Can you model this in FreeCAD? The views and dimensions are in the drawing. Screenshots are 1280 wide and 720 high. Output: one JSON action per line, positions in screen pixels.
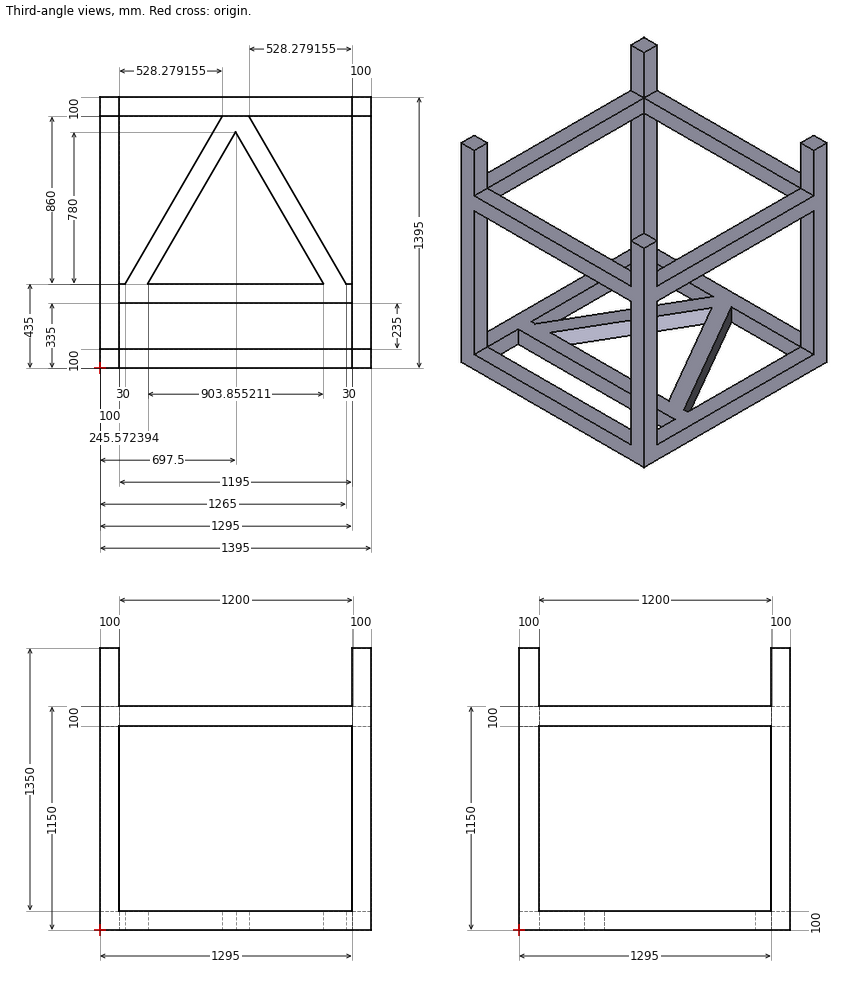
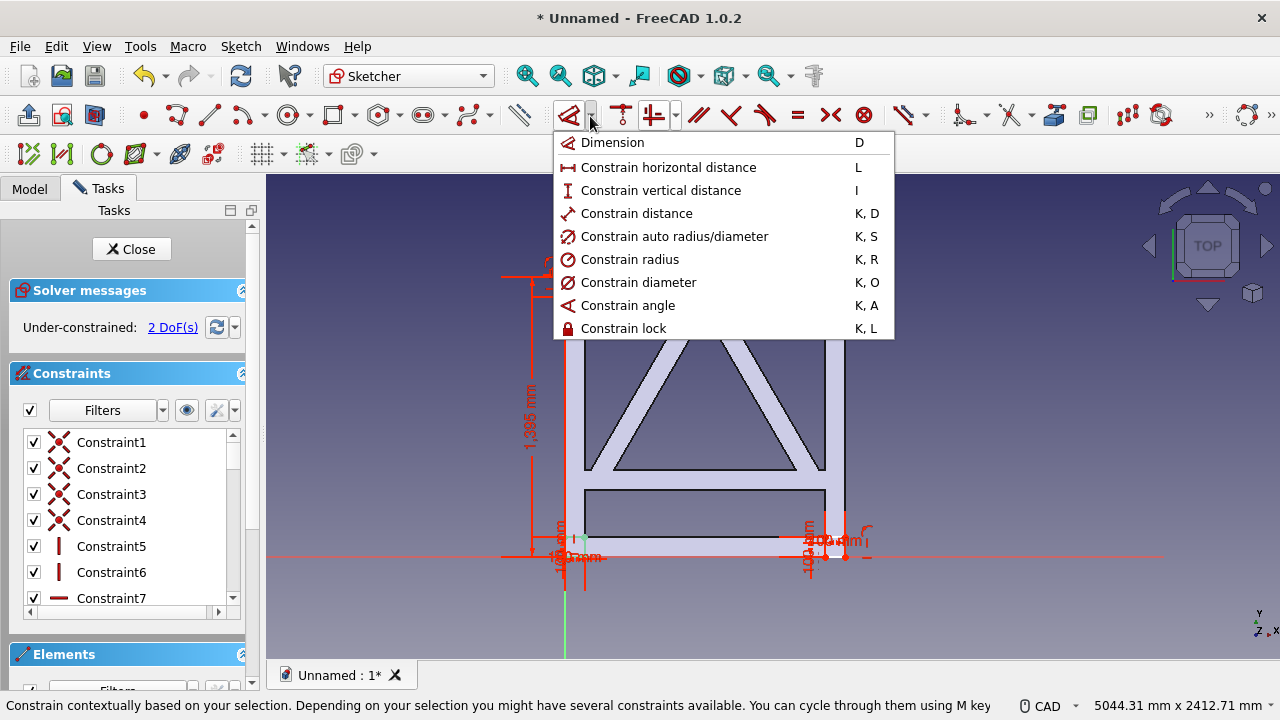
{"action": "left_click", "coordinate": [724, 190]}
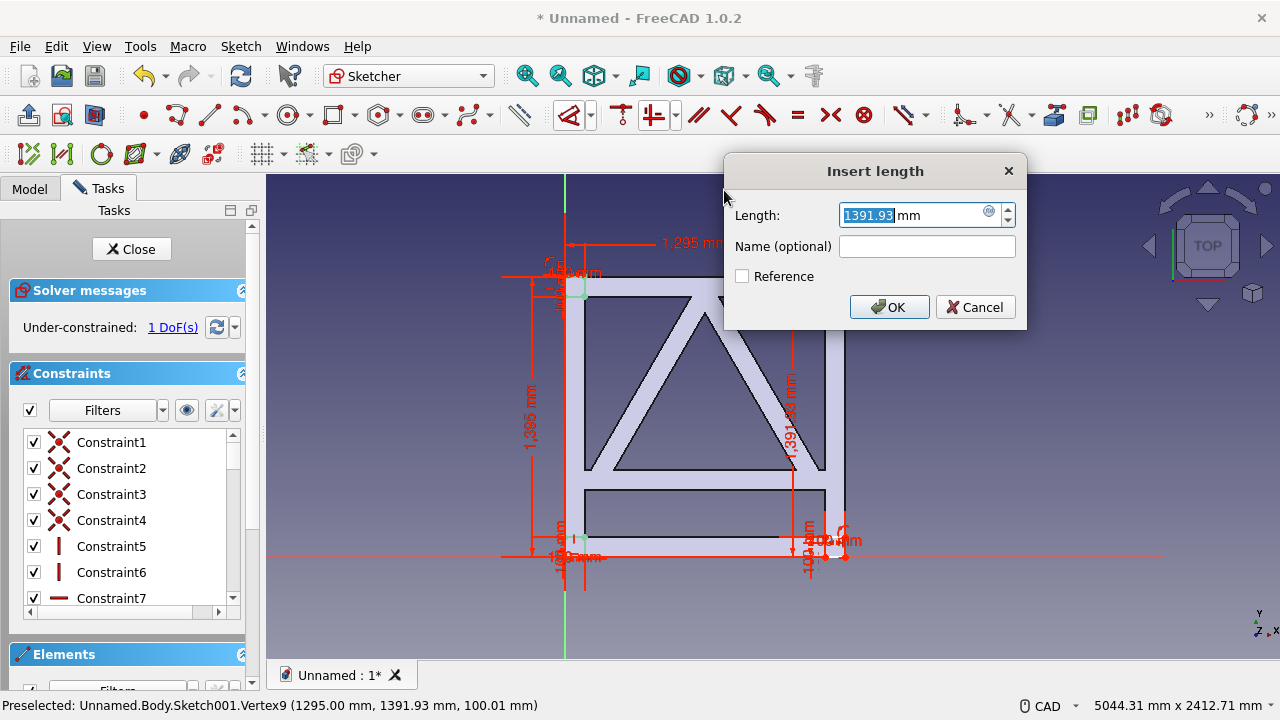
{"action": "type", "text": "1395"}
{"action": "key", "text": "Return"}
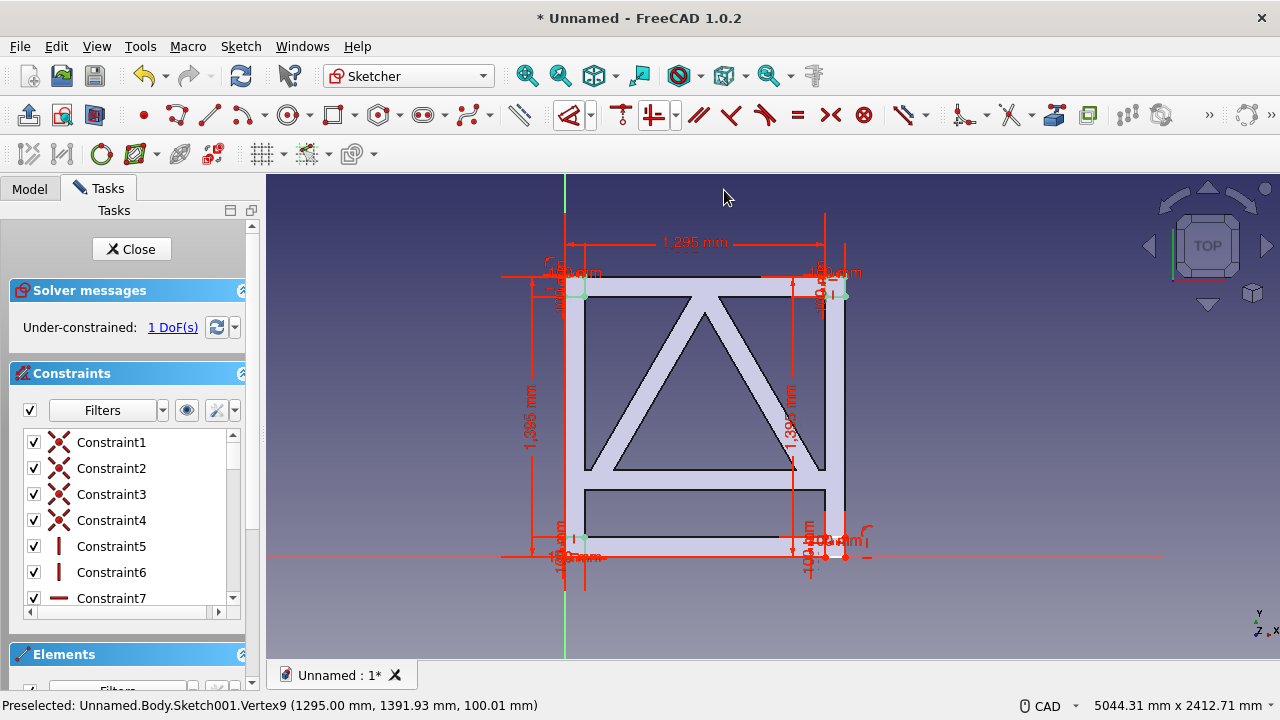
{"action": "left_click", "coordinate": [825, 537]}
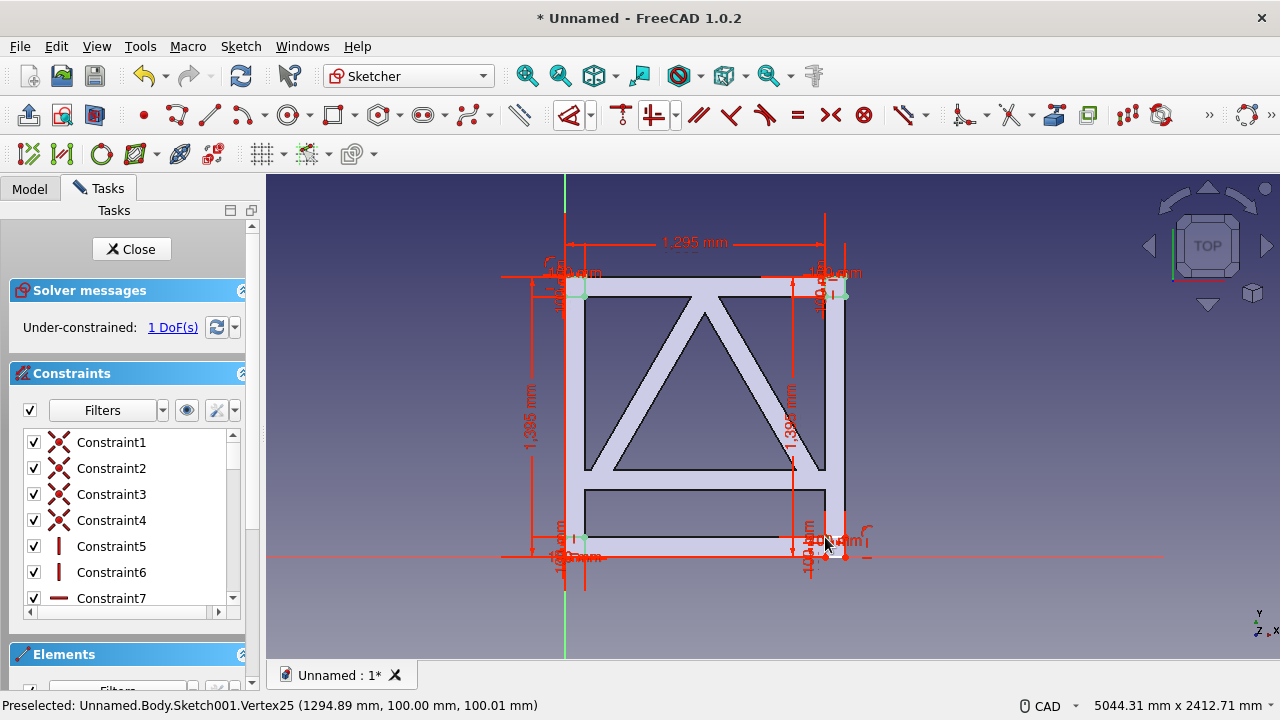
{"action": "left_click", "coordinate": [590, 116]}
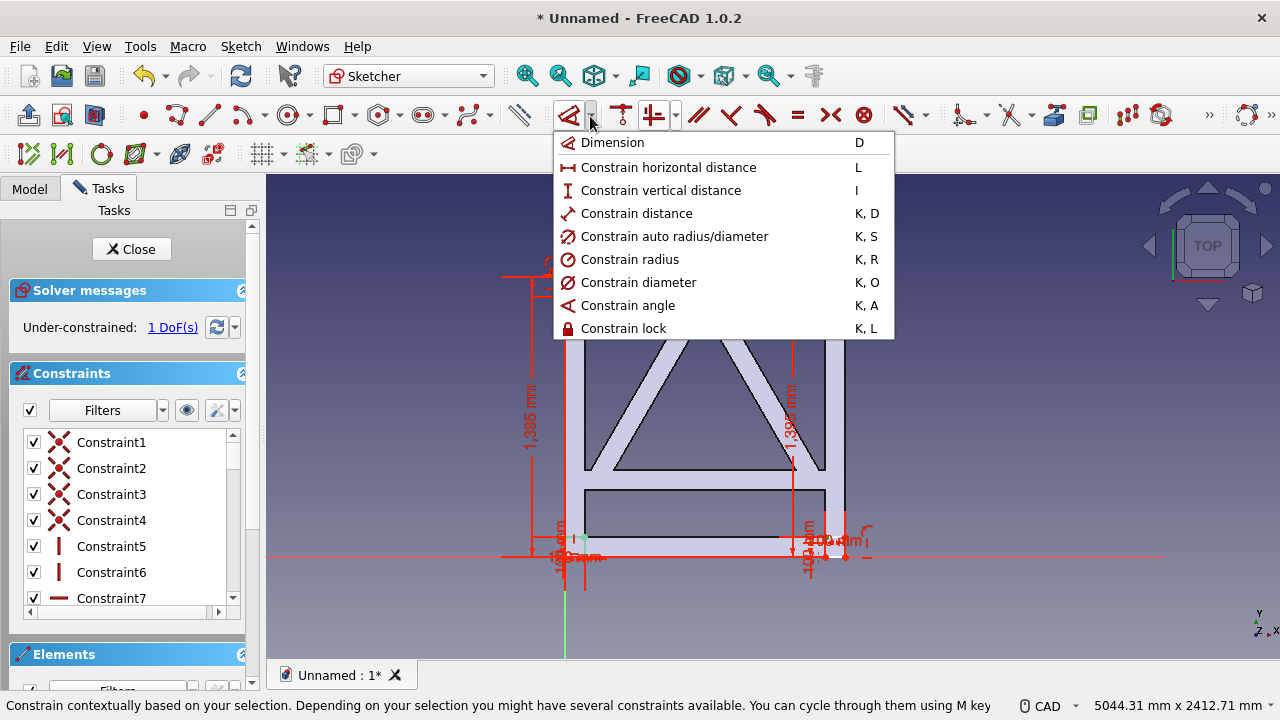
{"action": "left_click", "coordinate": [724, 168]}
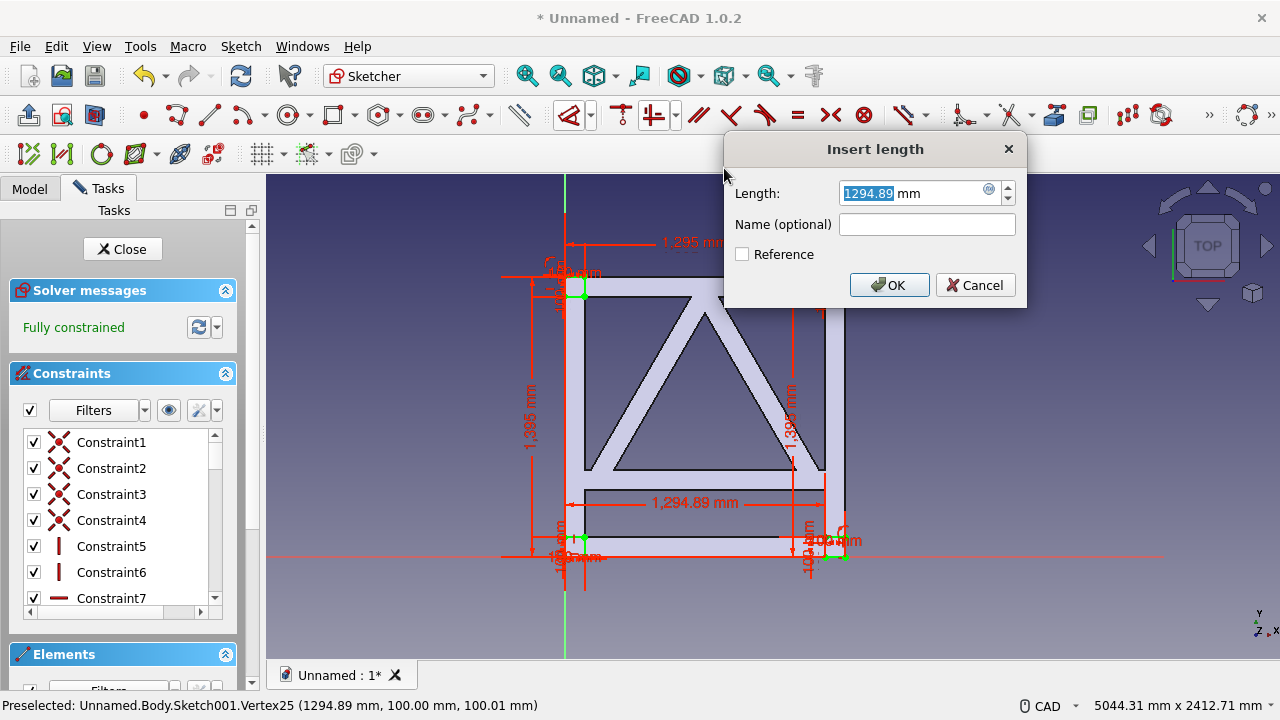
{"action": "type", "text": "1295"}
{"action": "key", "text": "Return"}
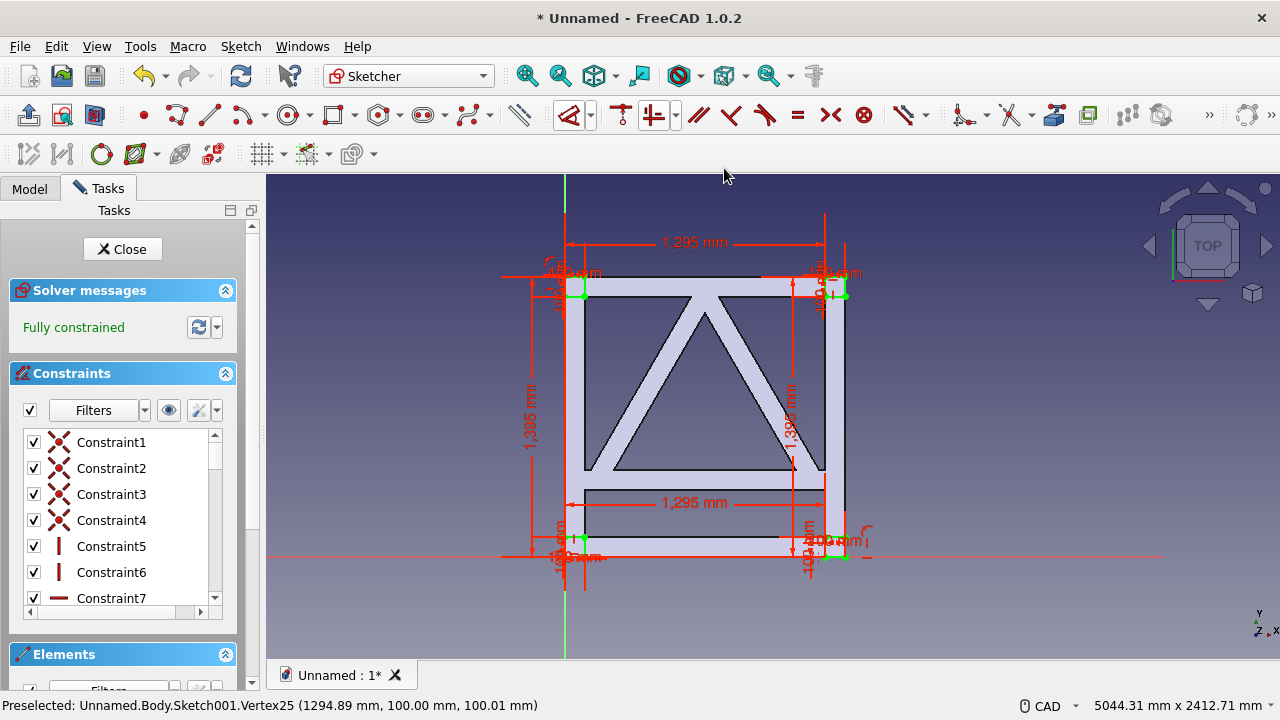
{"action": "left_click", "coordinate": [123, 249]}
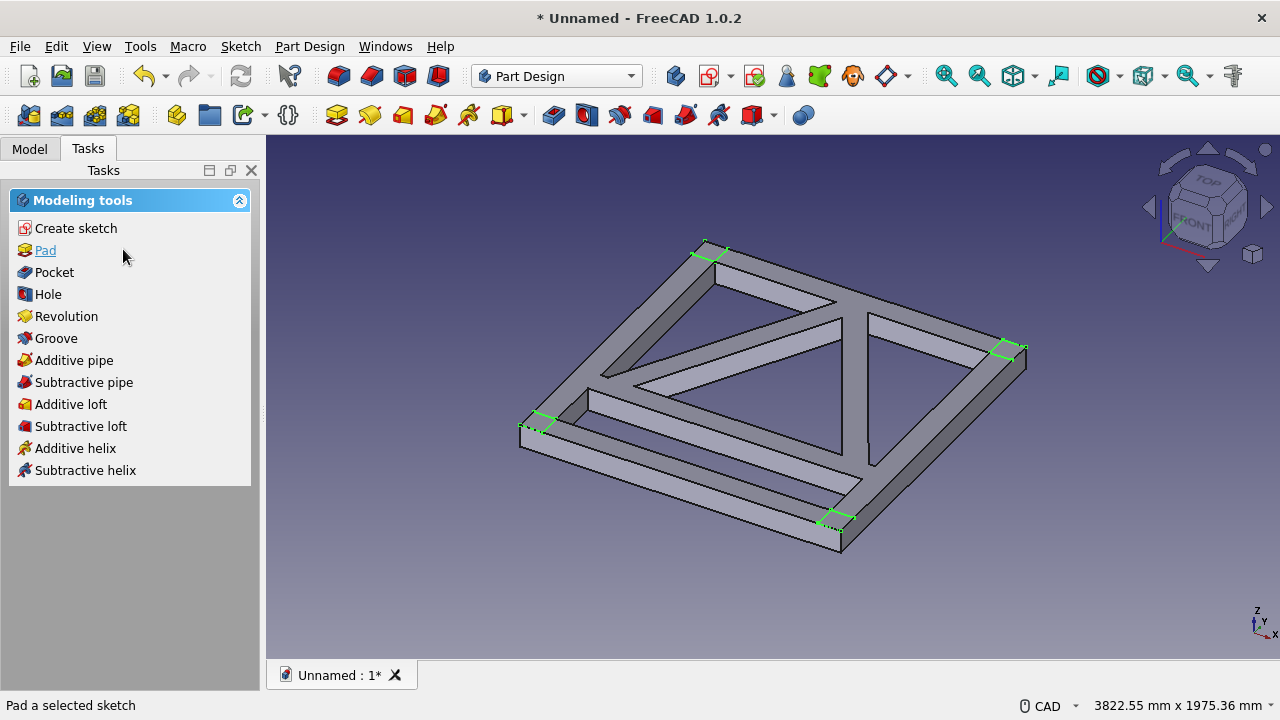
{"action": "left_click", "coordinate": [337, 116]}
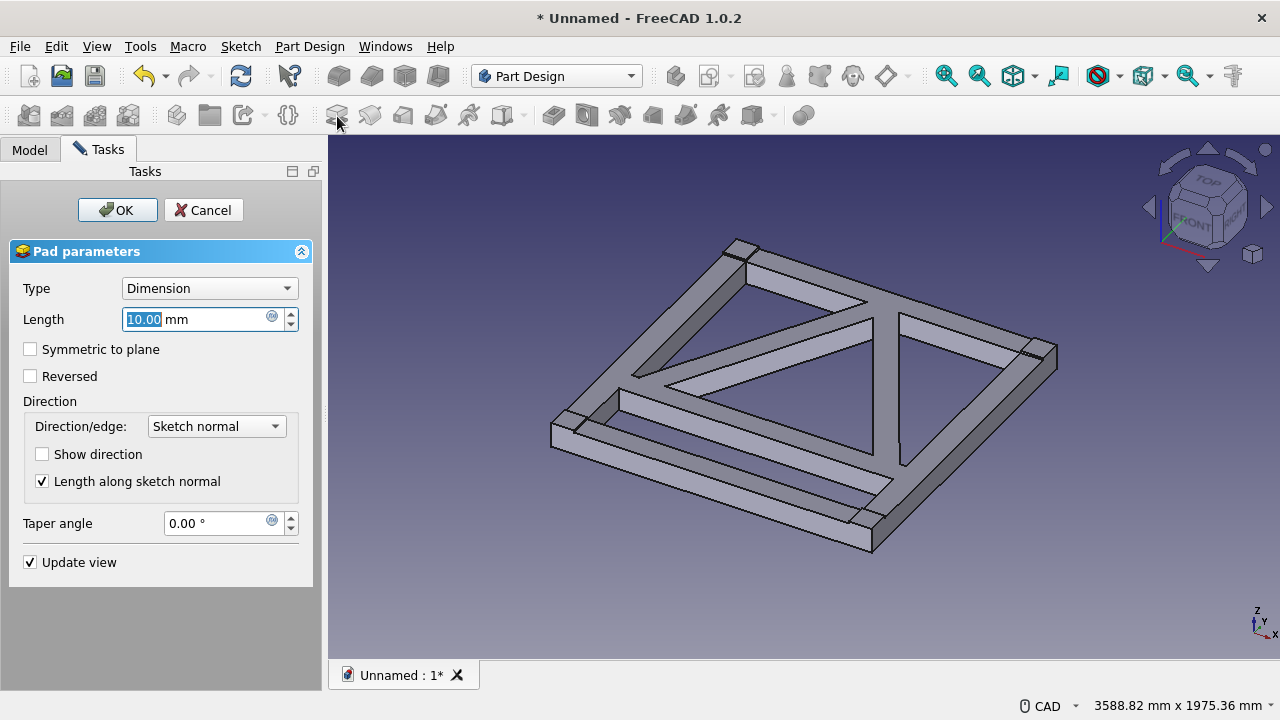
{"action": "type", "text": "1350"}
{"action": "key", "text": "Tab"}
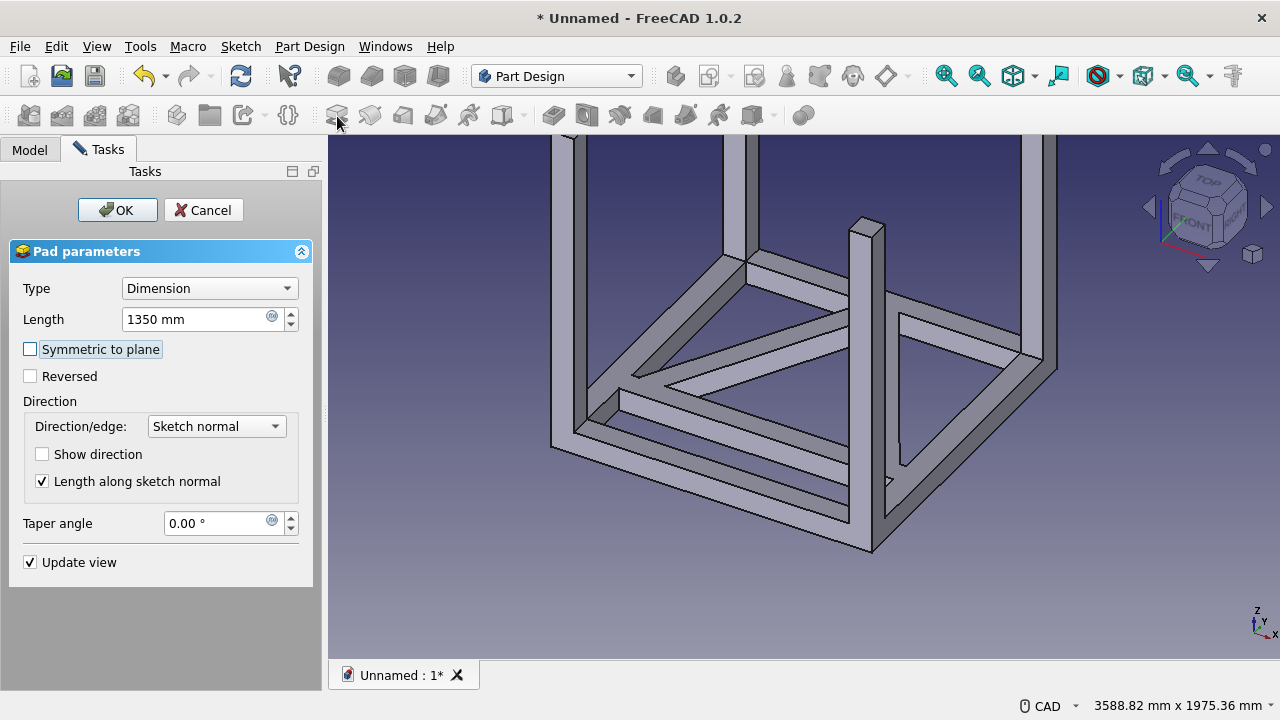
{"action": "left_click", "coordinate": [118, 210]}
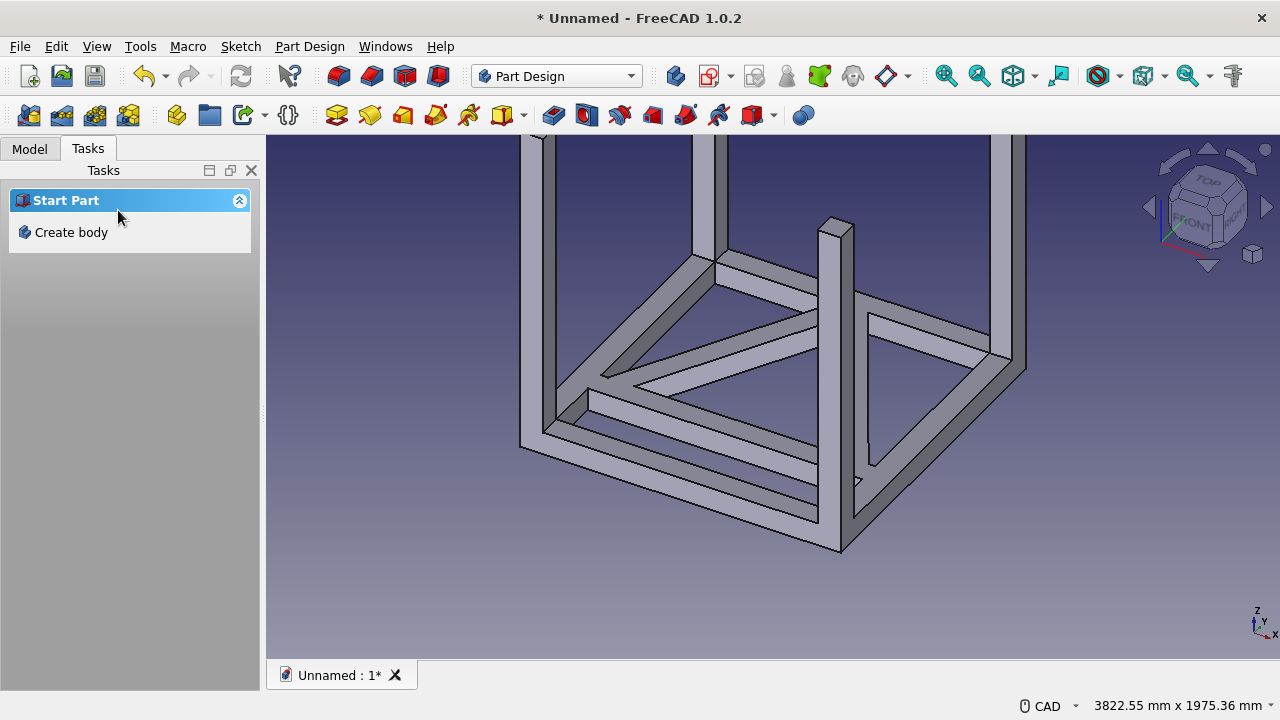
{"action": "left_click", "coordinate": [947, 76]}